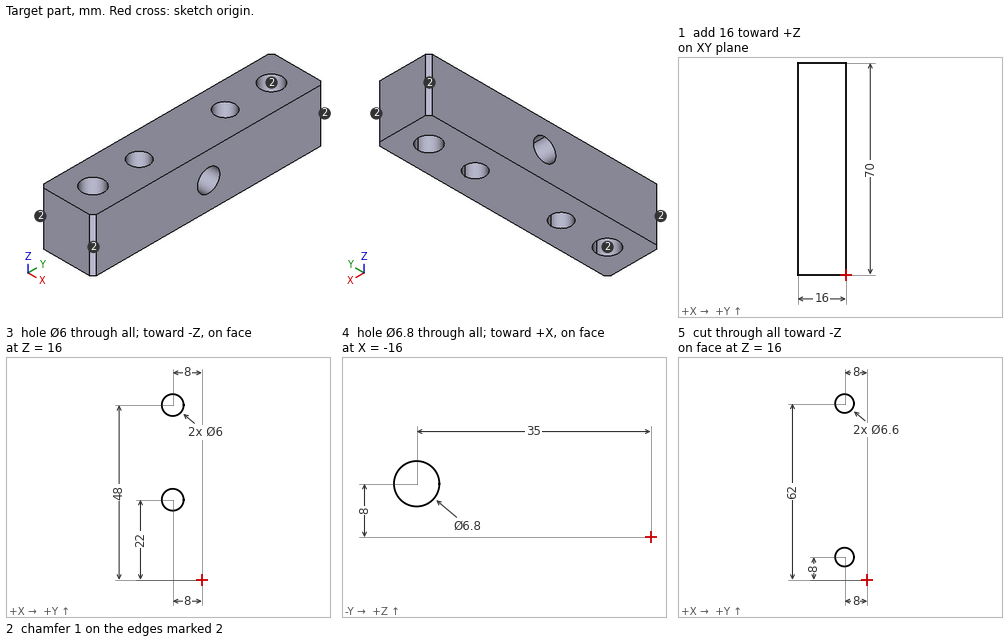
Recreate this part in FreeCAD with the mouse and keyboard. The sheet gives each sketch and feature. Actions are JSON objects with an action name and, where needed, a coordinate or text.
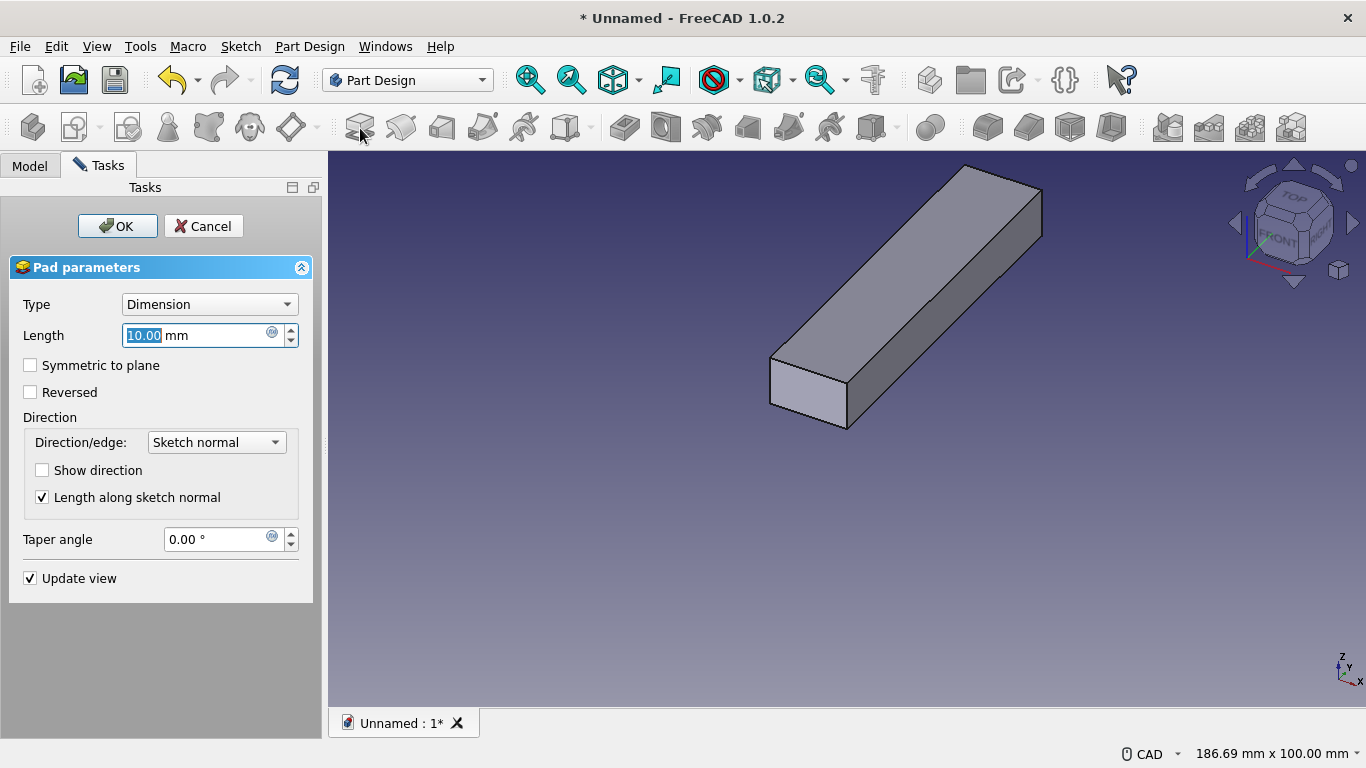
{"action": "type", "text": "16"}
{"action": "key", "text": "Tab"}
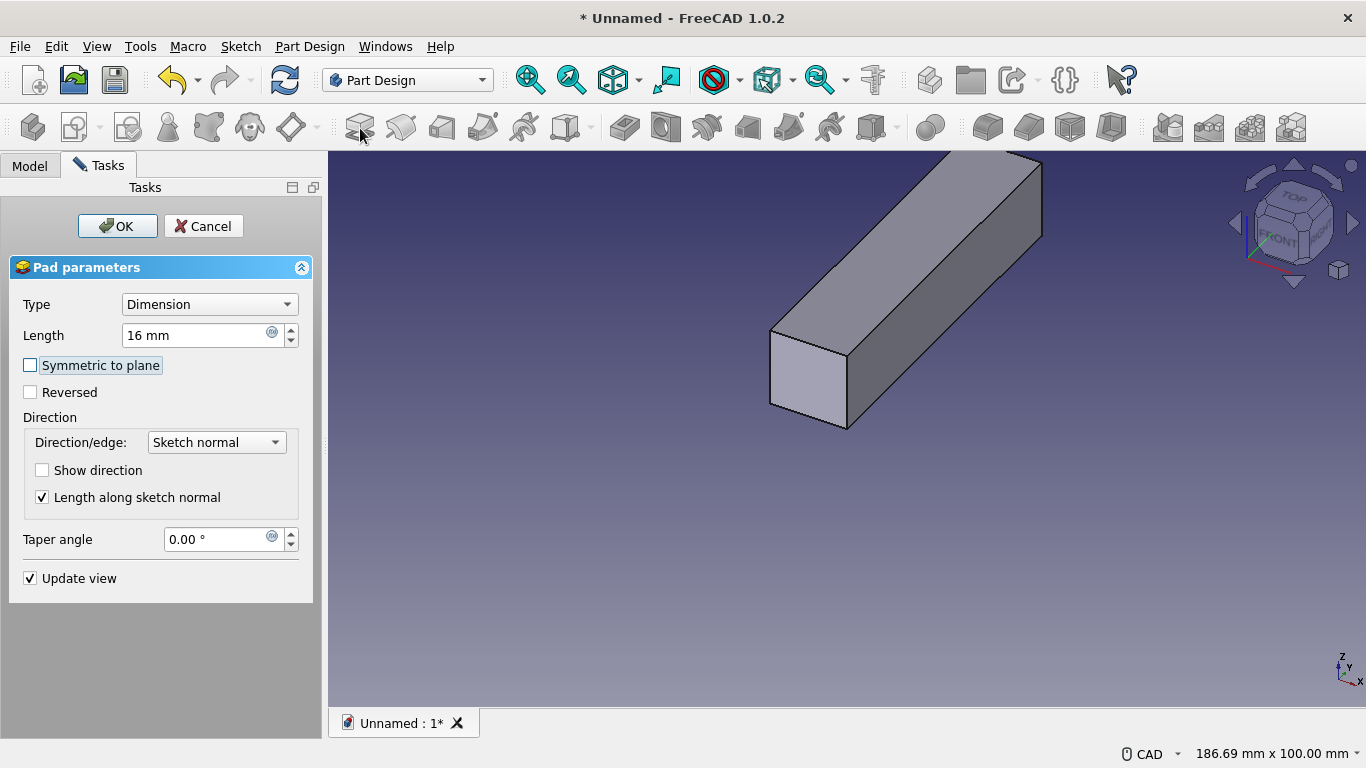
{"action": "left_click", "coordinate": [118, 226]}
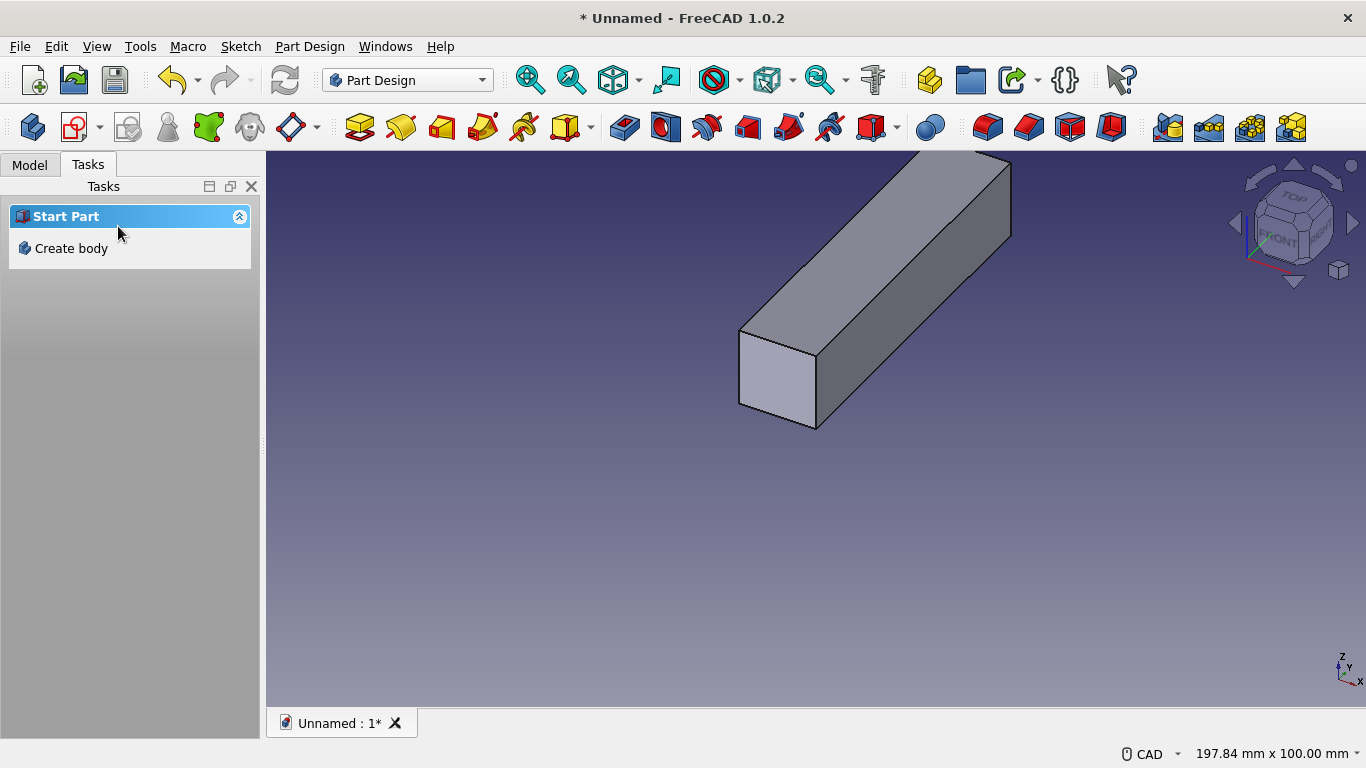
{"action": "left_click", "coordinate": [531, 80]}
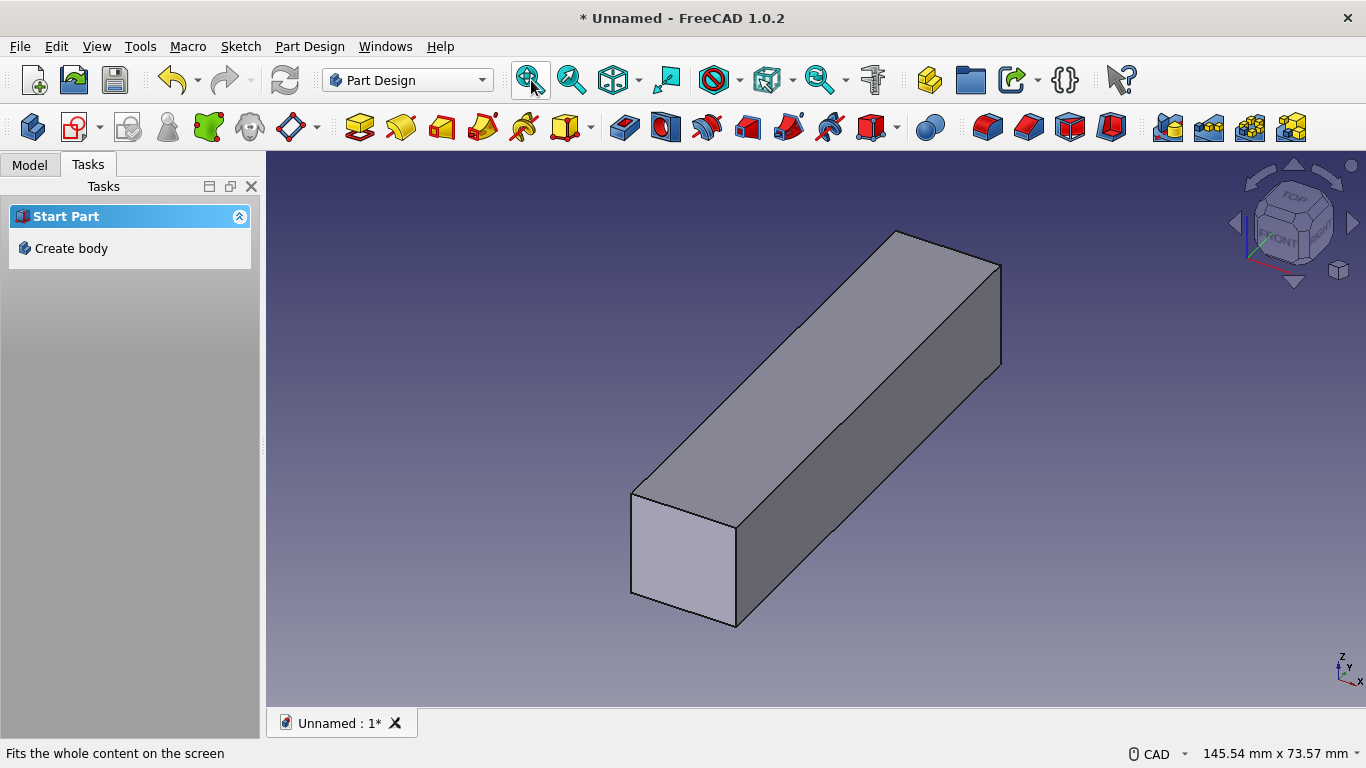
{"action": "left_click", "coordinate": [736, 577]}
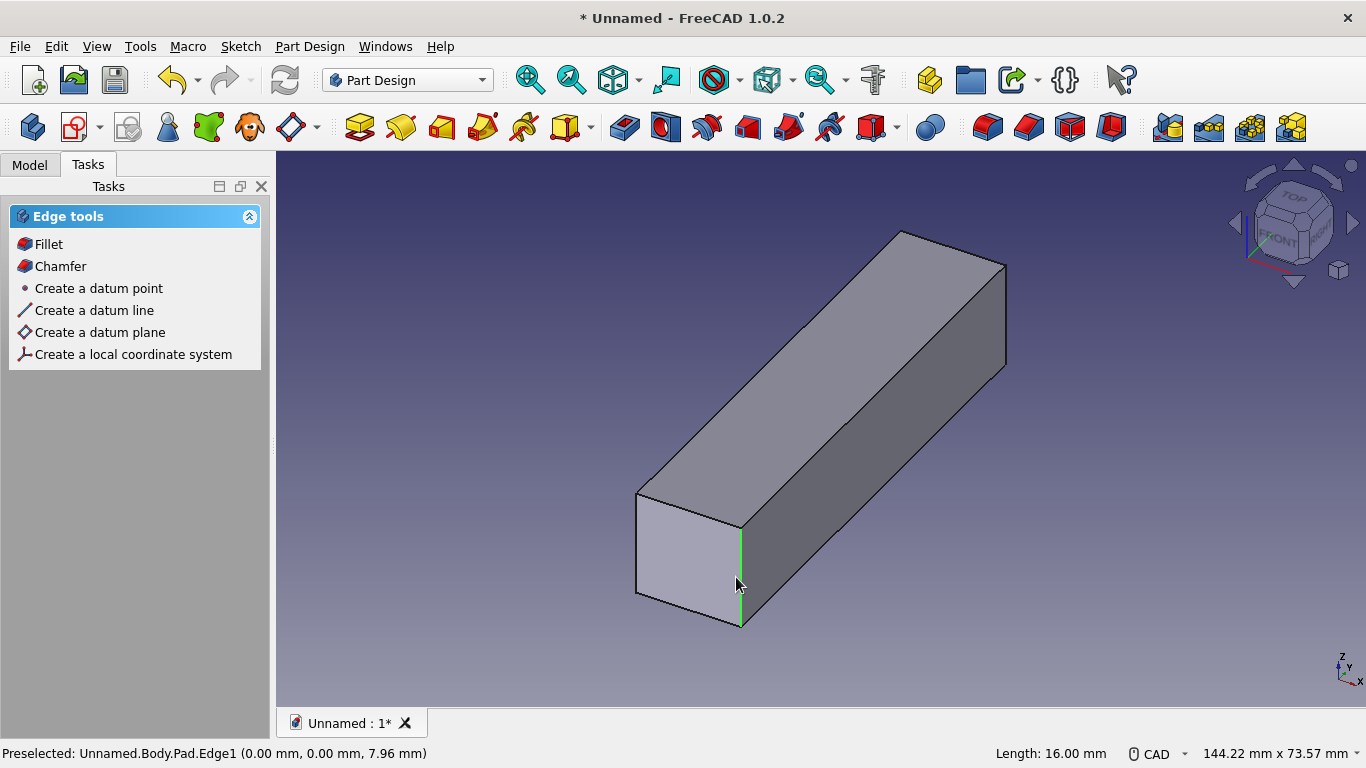
{"action": "key", "text": "0"}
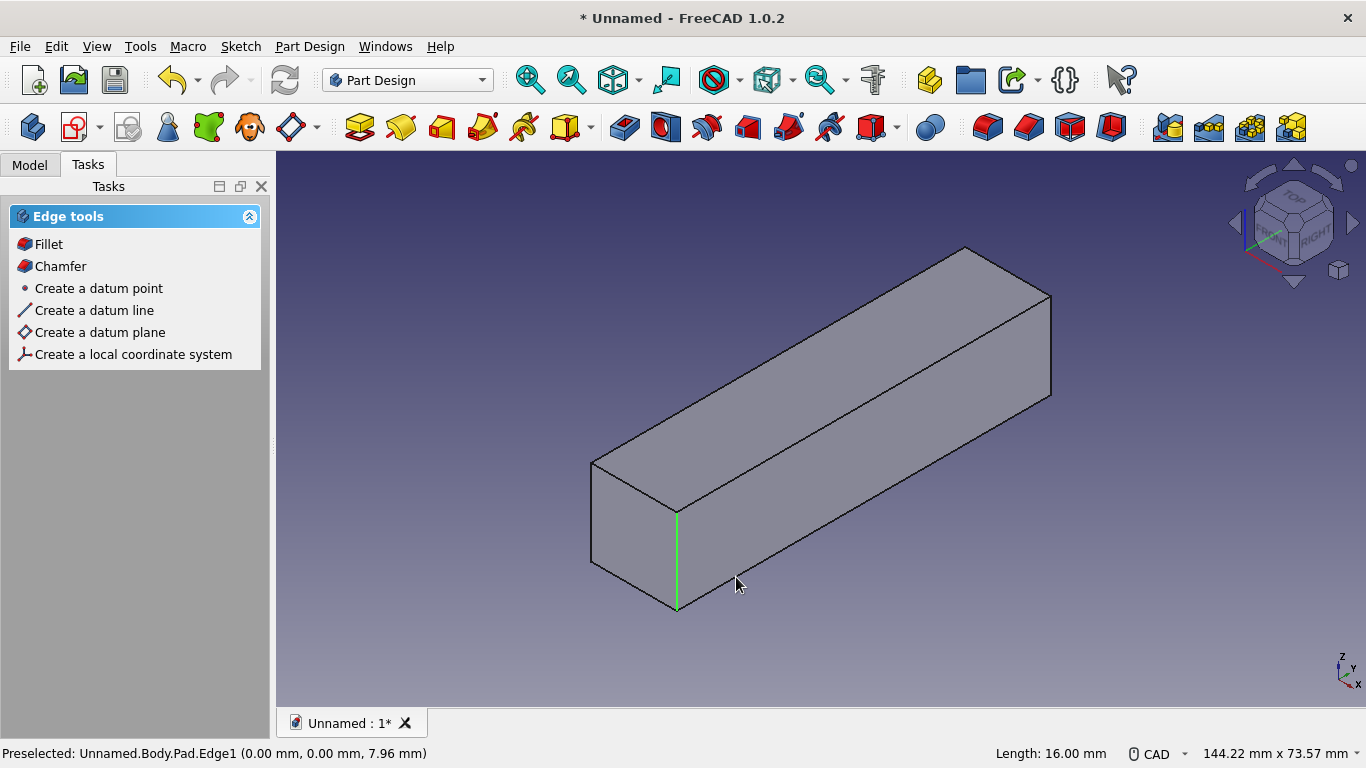
{"action": "key", "text": "2"}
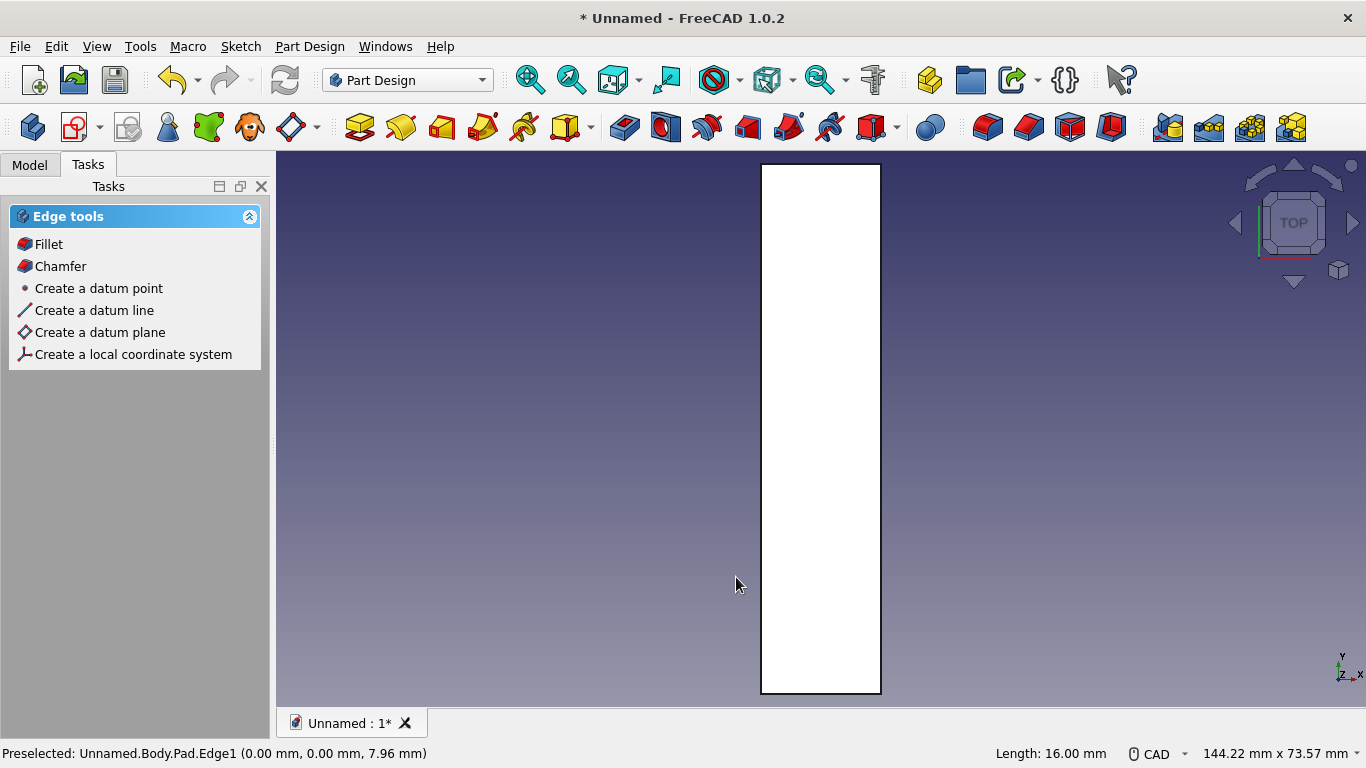
{"action": "key", "text": "1"}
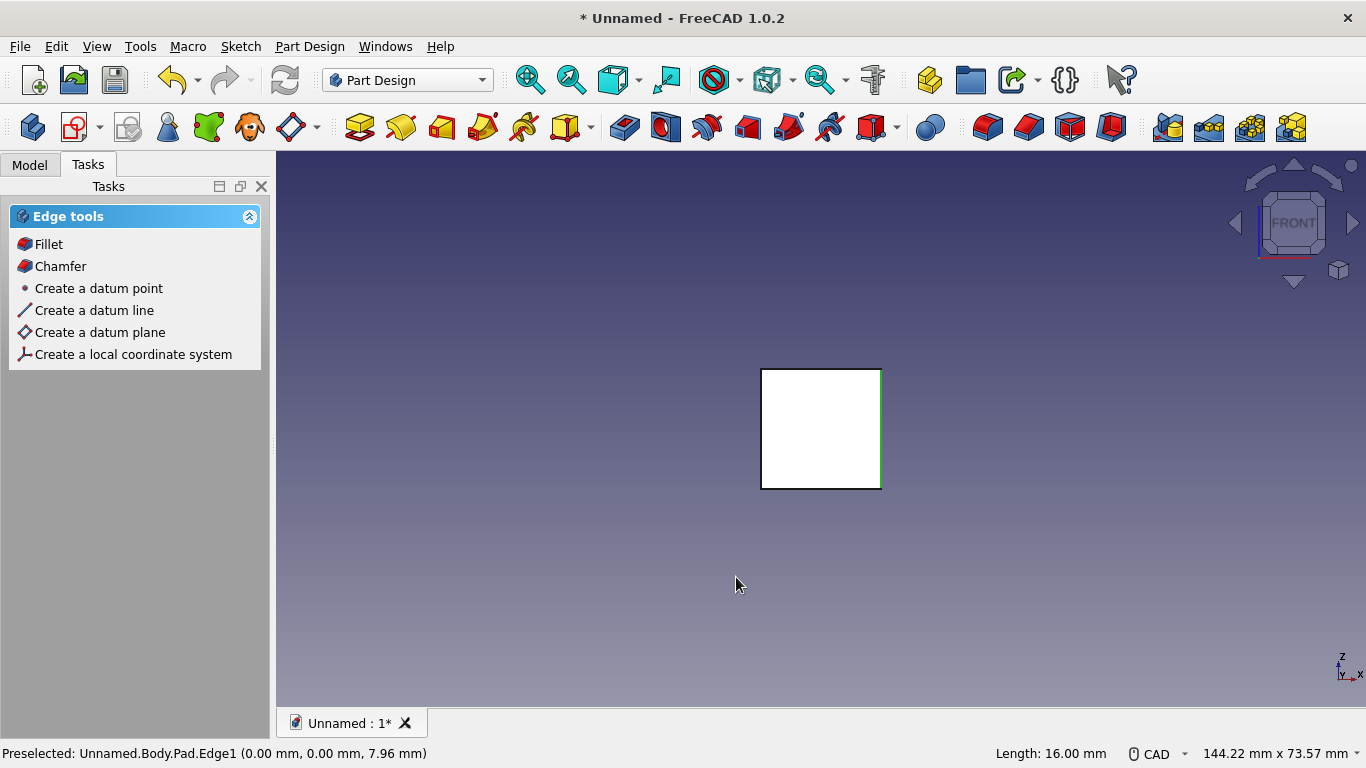
{"action": "left_click", "coordinate": [531, 80]}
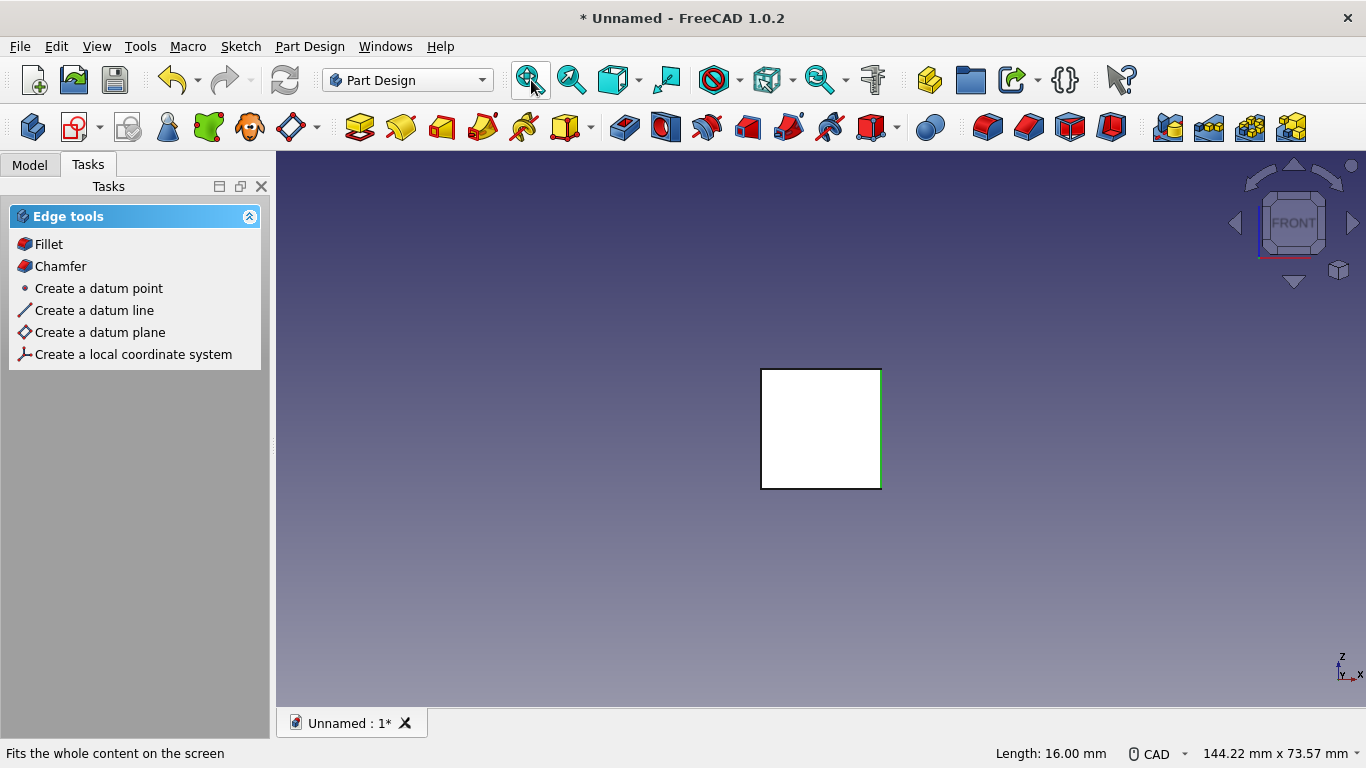
{"action": "left_click", "coordinate": [761, 428], "text": "ctrl"}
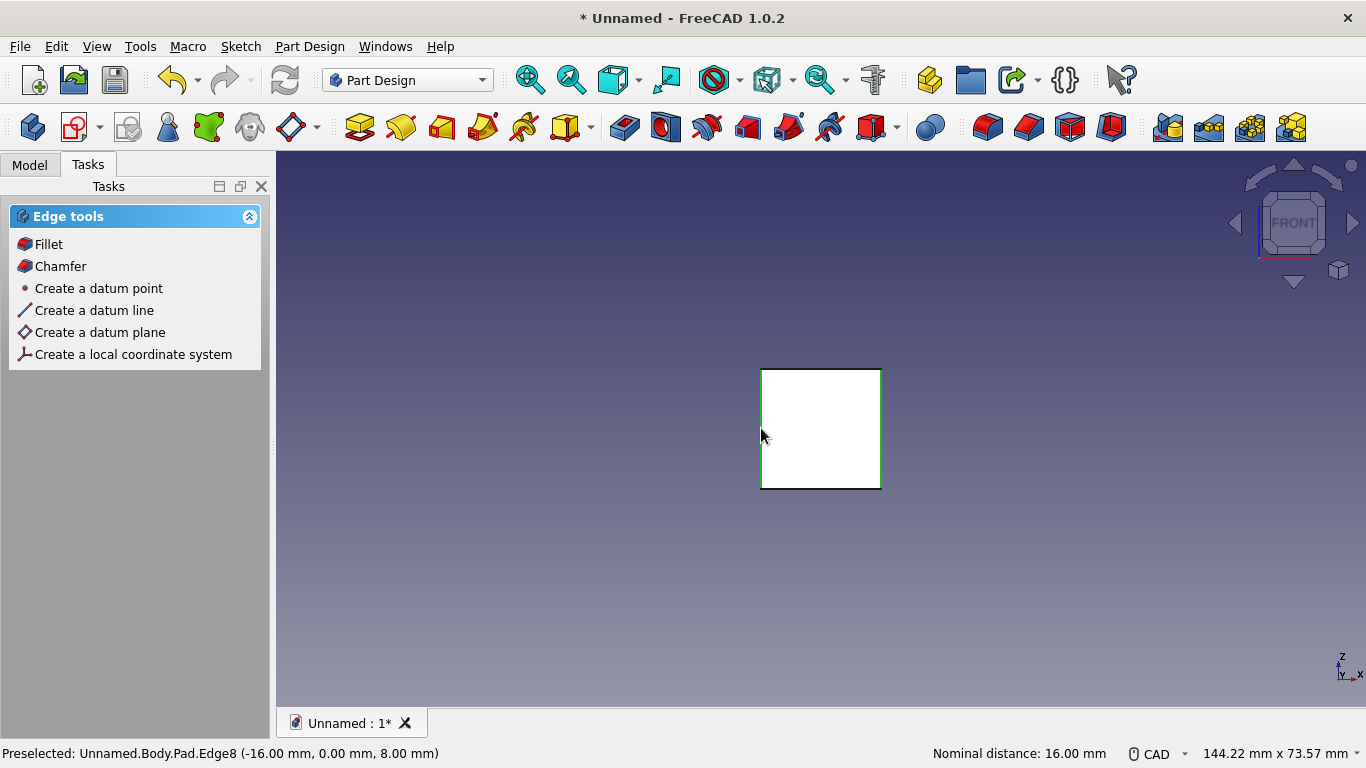
{"action": "key", "text": "3"}